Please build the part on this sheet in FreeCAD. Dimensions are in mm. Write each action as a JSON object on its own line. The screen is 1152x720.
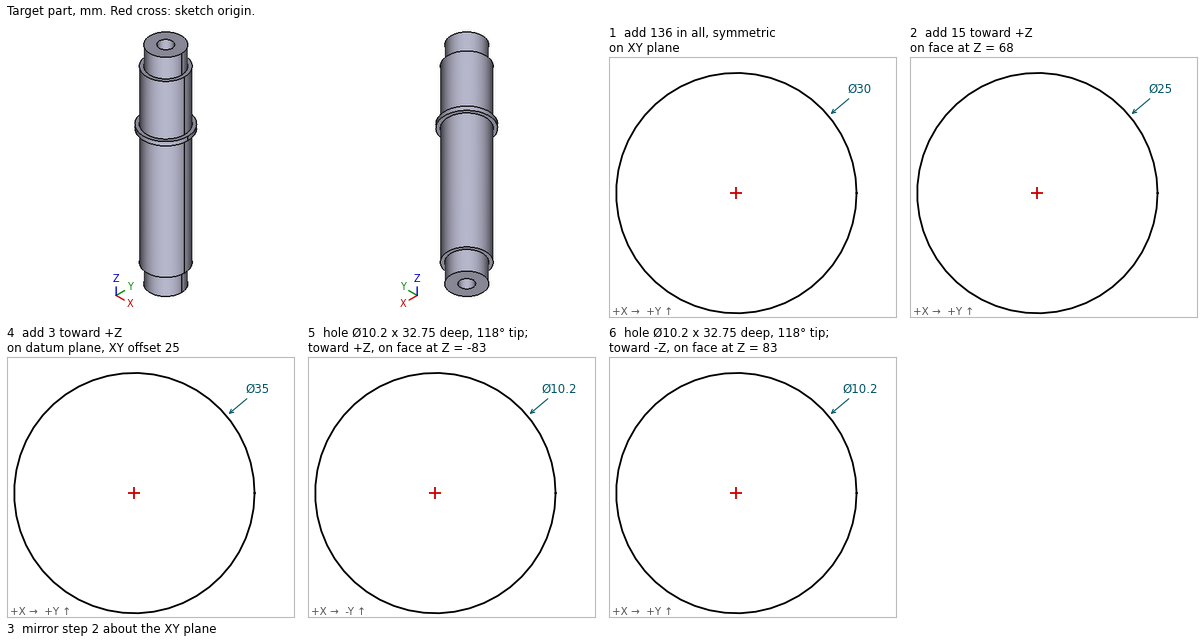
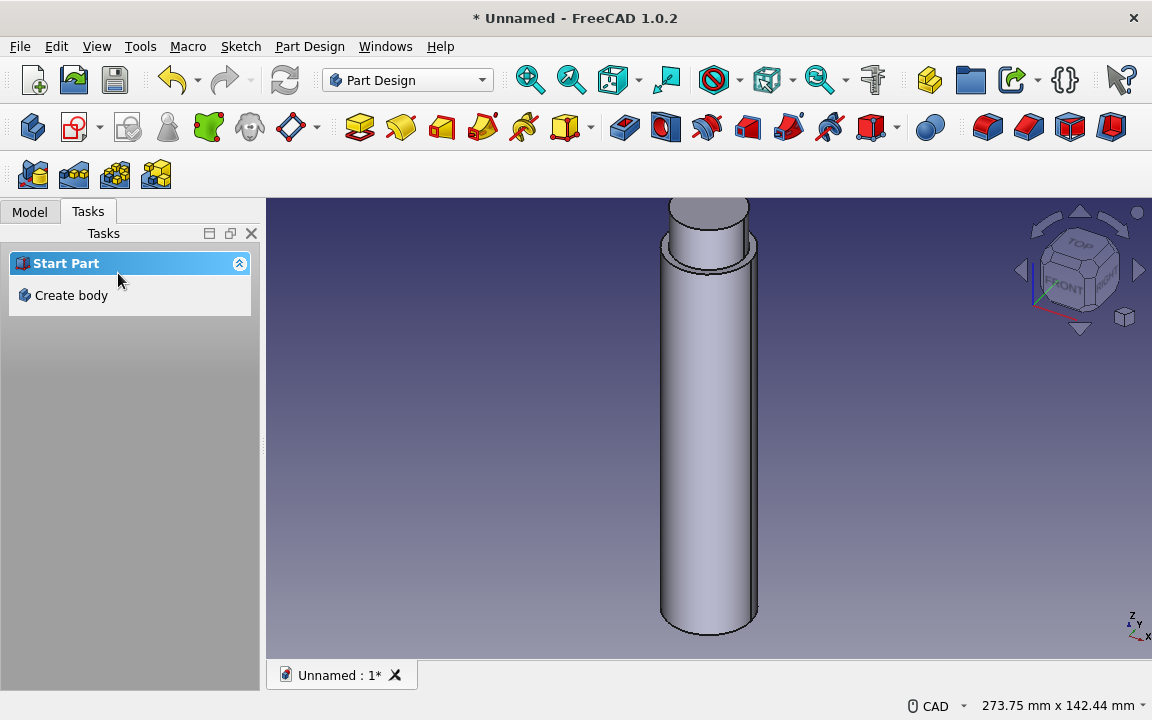
{"action": "left_click", "coordinate": [531, 80]}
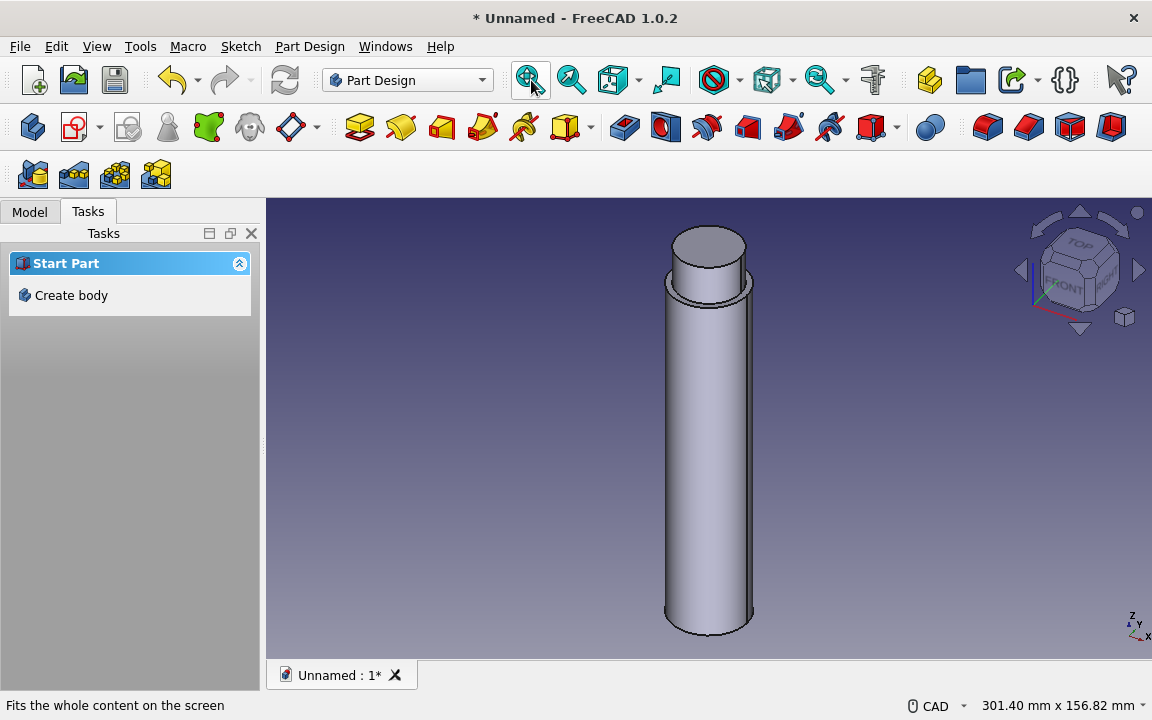
{"action": "left_click", "coordinate": [30, 212]}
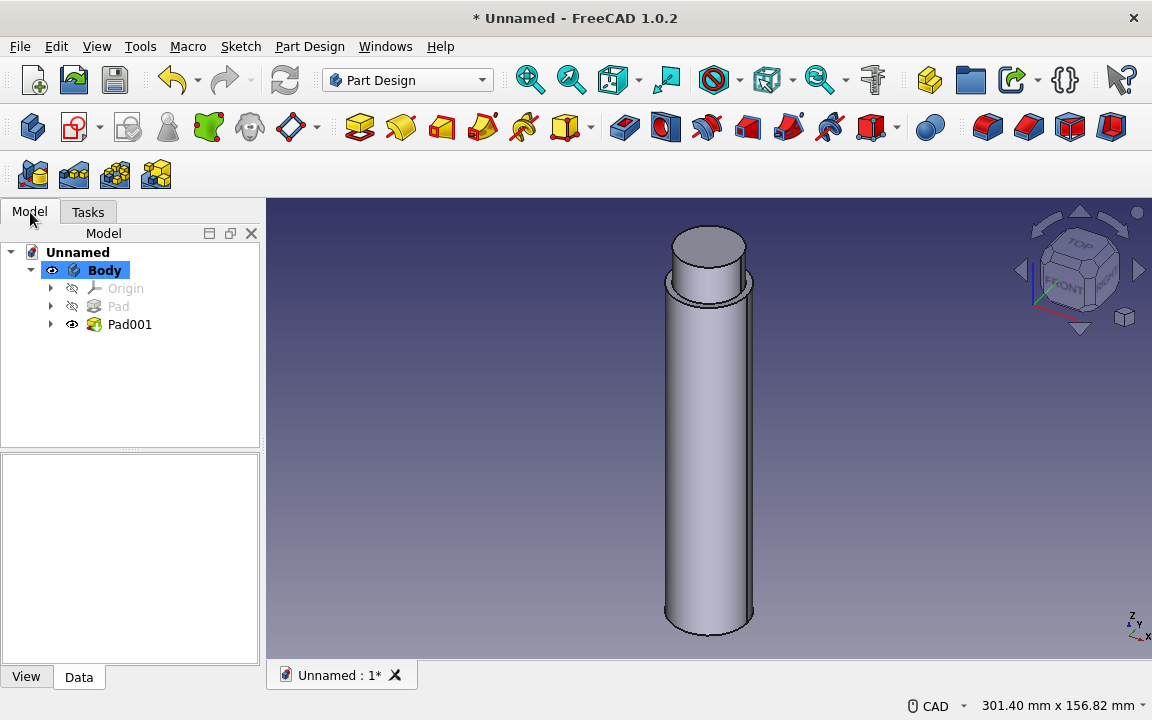
{"action": "left_click", "coordinate": [117, 324]}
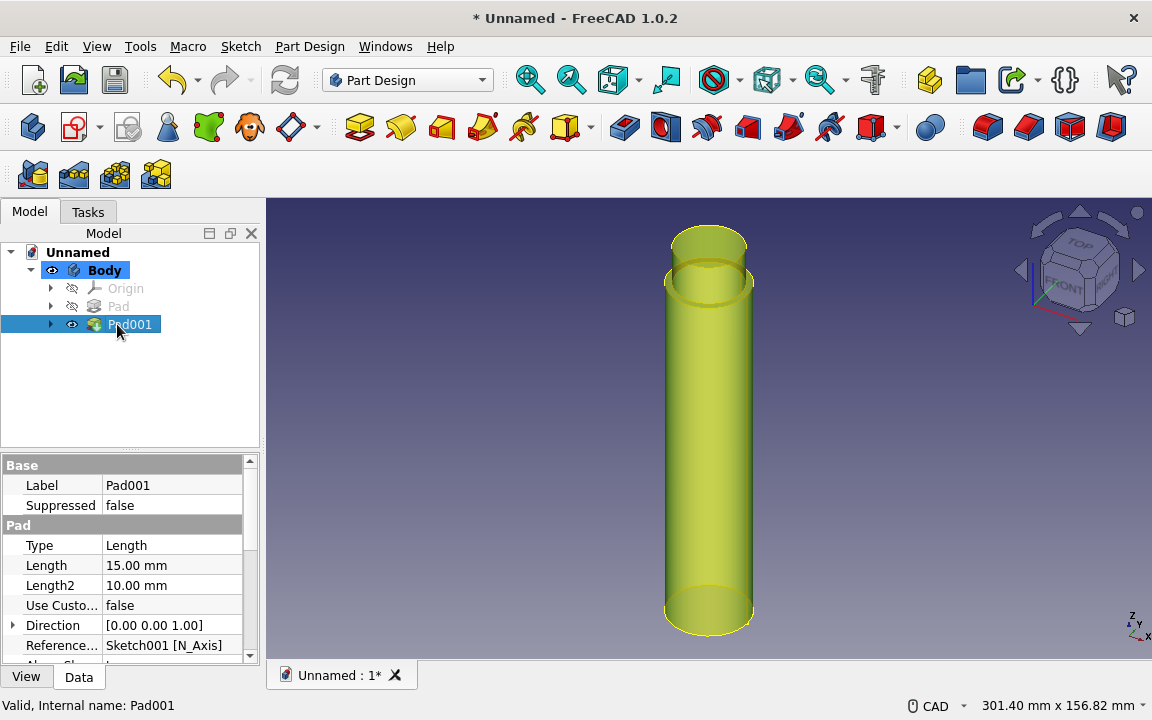
{"action": "left_click", "coordinate": [33, 174]}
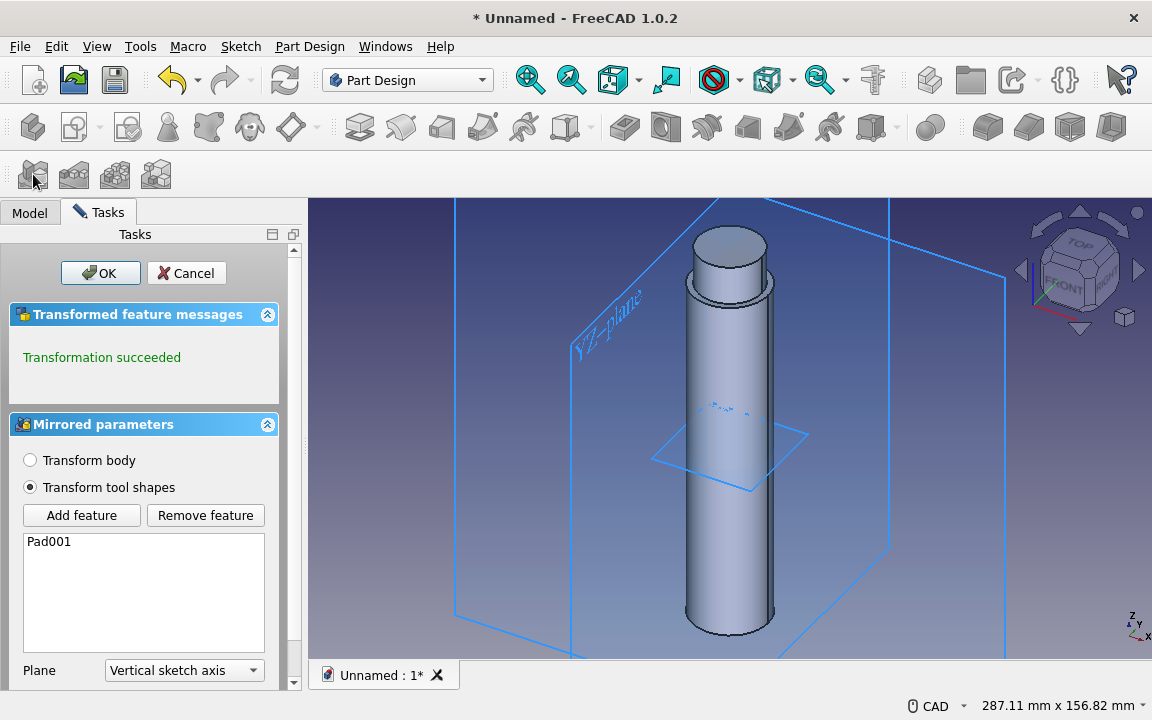
{"action": "left_click", "coordinate": [185, 670]}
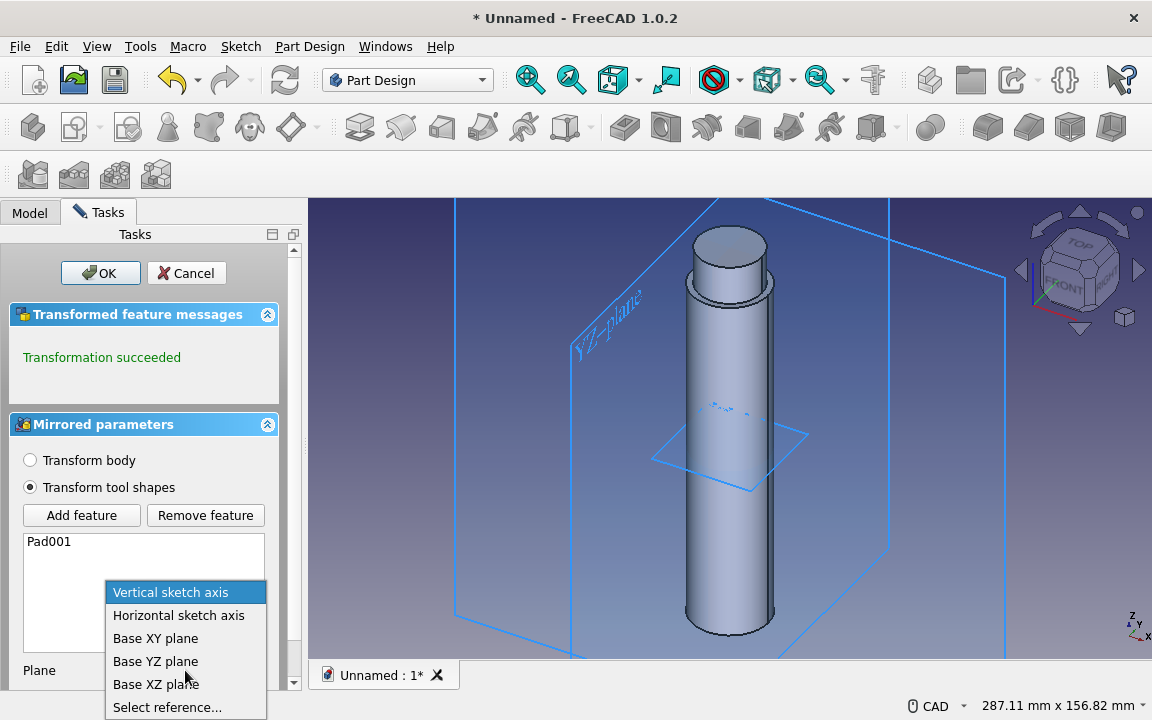
{"action": "left_click", "coordinate": [184, 638]}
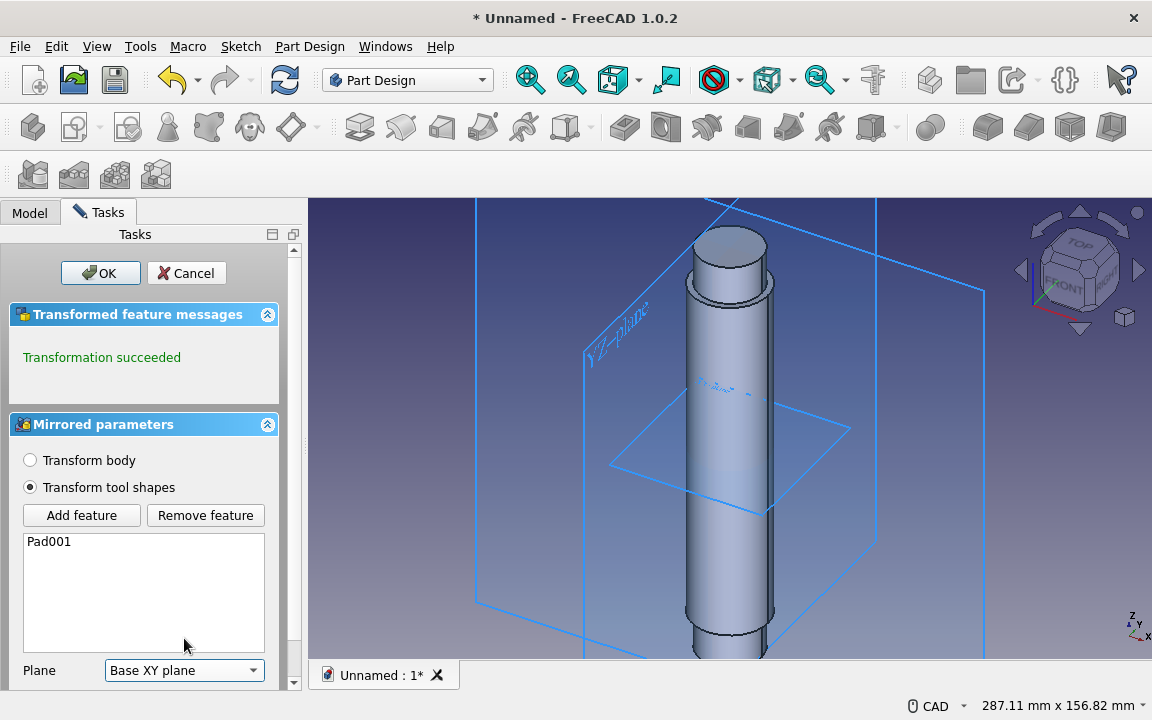
{"action": "left_click", "coordinate": [101, 273]}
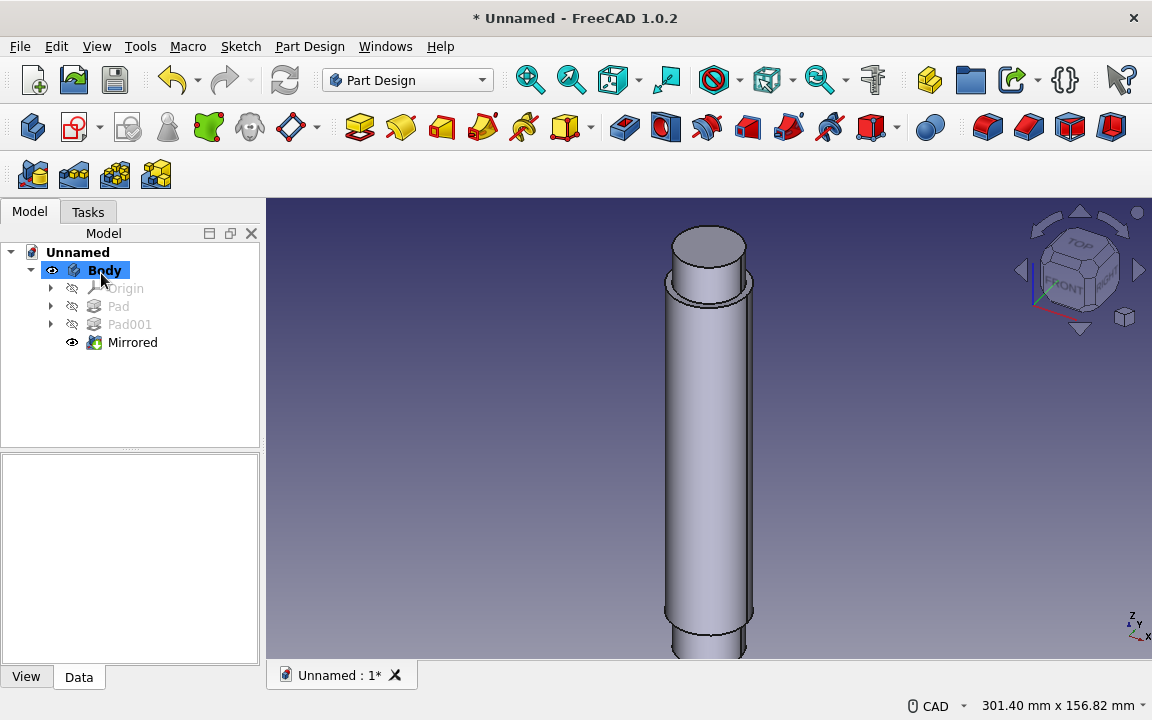
{"action": "left_click", "coordinate": [531, 80]}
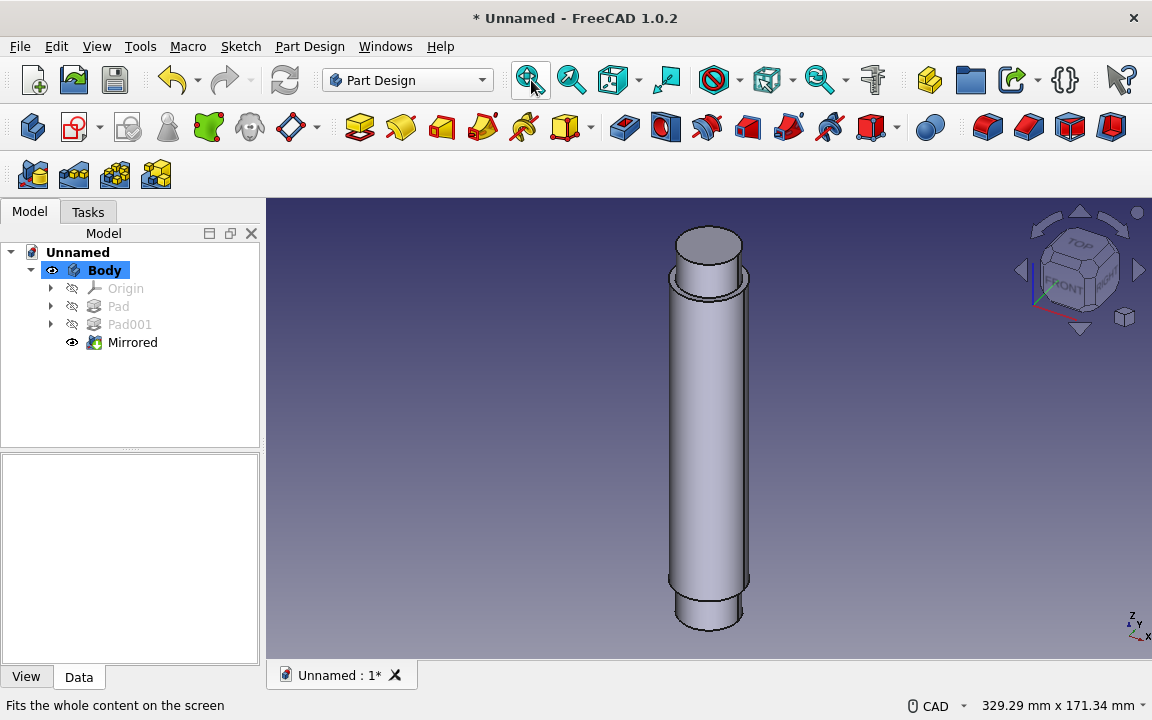
{"action": "left_click", "coordinate": [51, 288]}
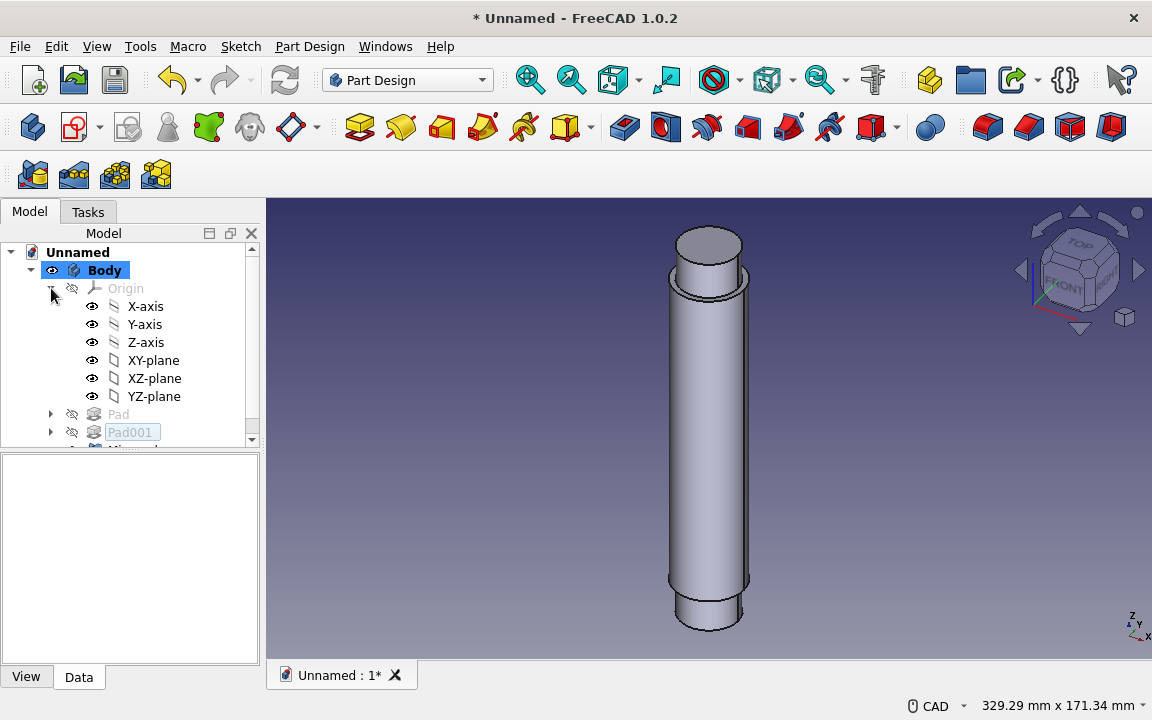
{"action": "left_click", "coordinate": [137, 360]}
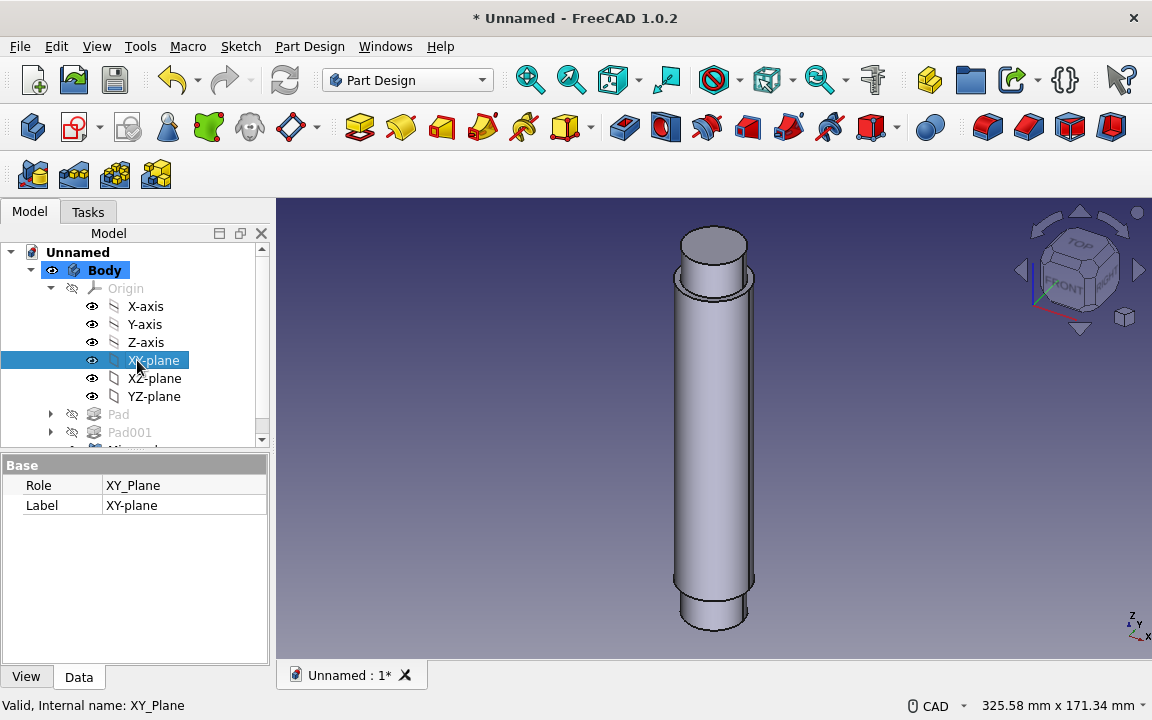
{"action": "left_click", "coordinate": [290, 128]}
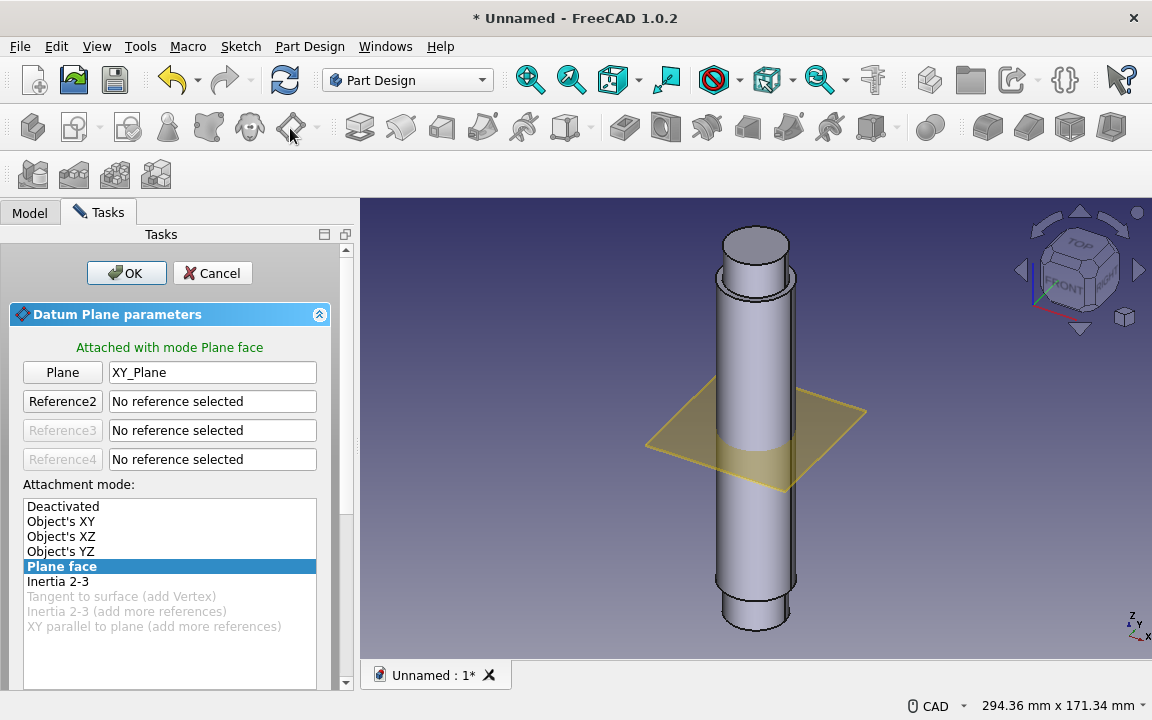
{"action": "scroll", "coordinate": [346, 467], "scroll_direction": "down", "scroll_amount": 4}